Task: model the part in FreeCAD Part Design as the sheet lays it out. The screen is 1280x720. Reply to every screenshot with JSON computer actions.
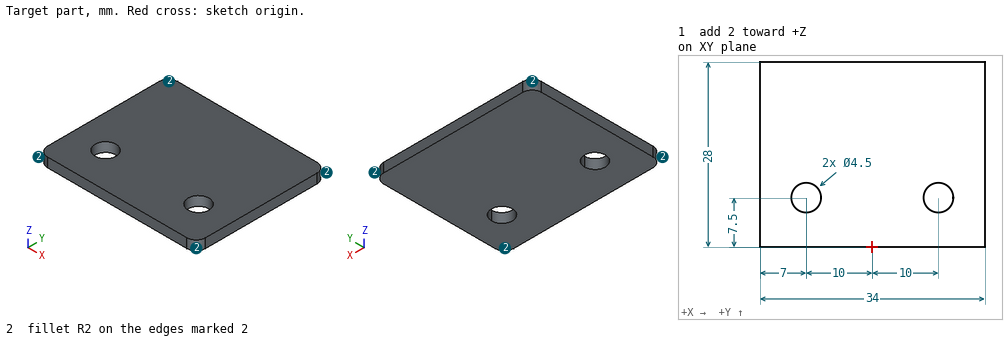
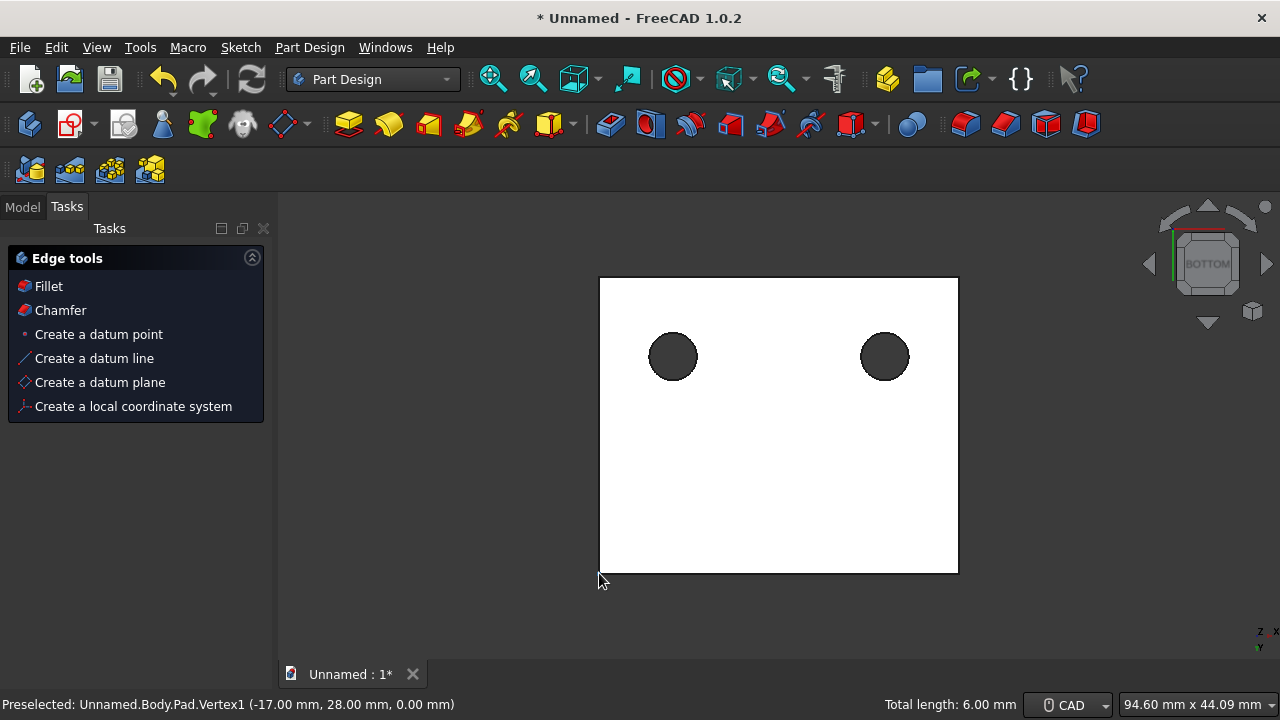
{"action": "key", "text": "4"}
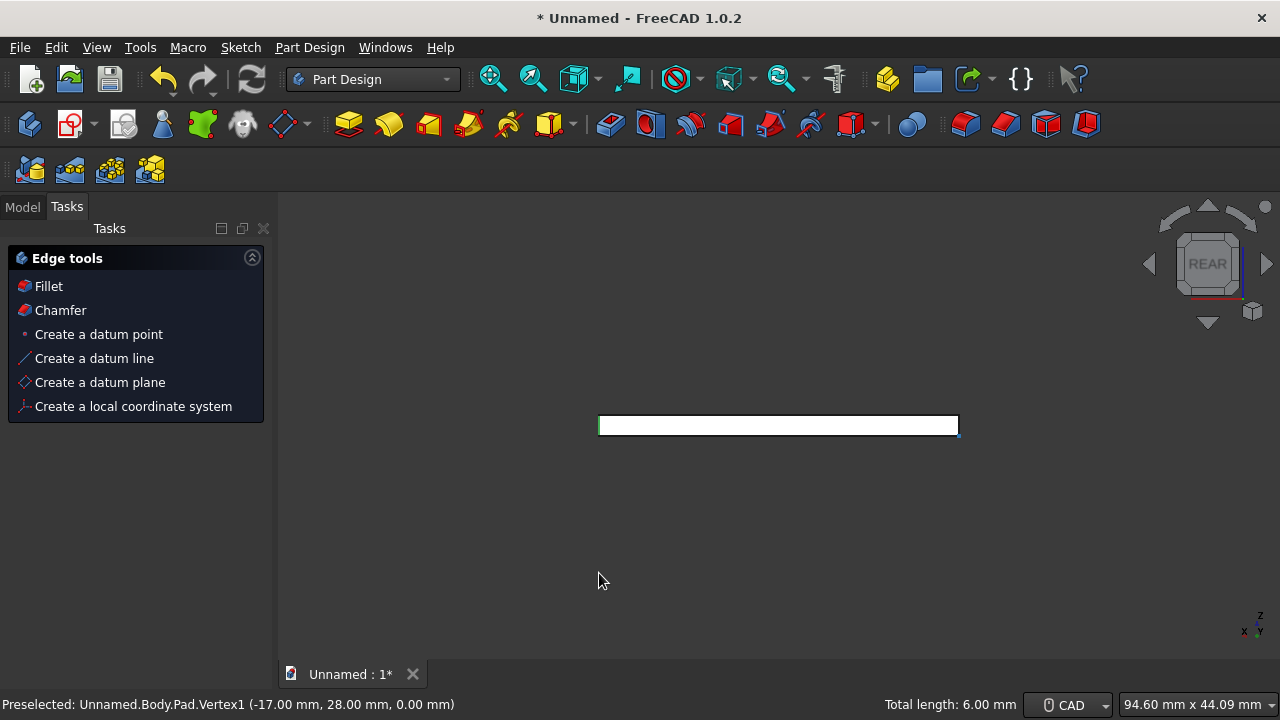
{"action": "key", "text": "v f"}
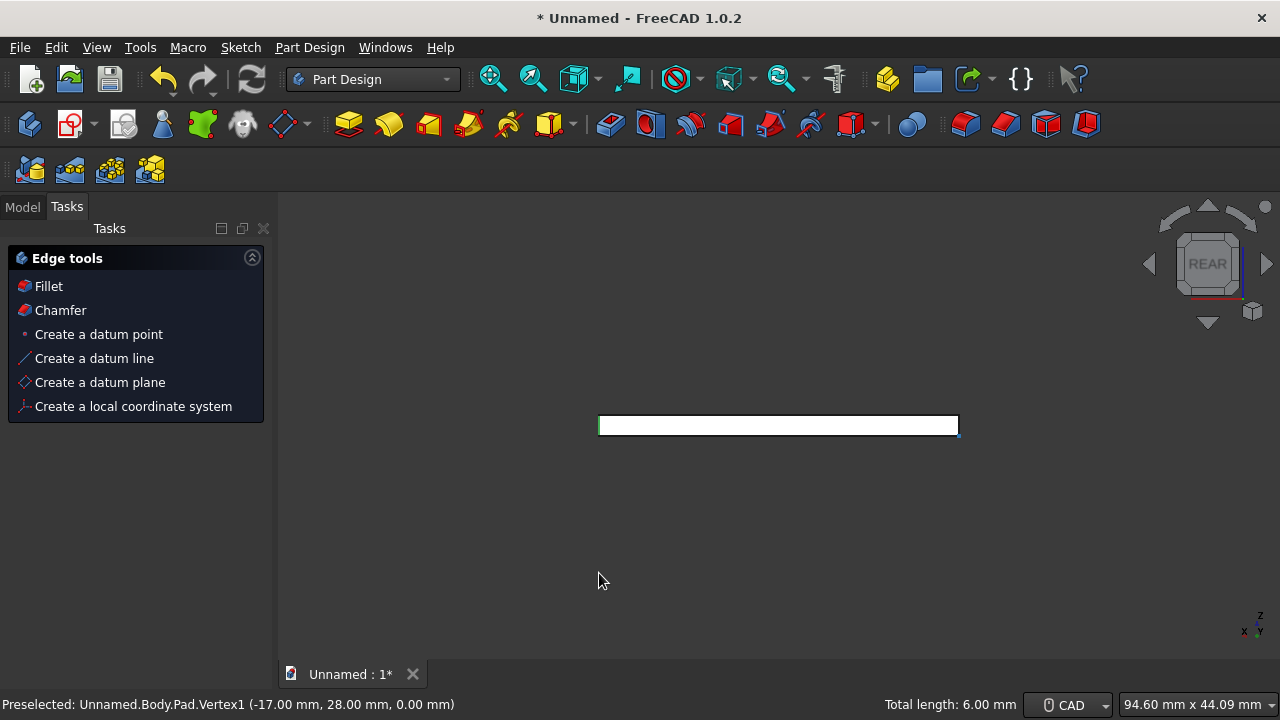
{"action": "left_click", "coordinate": [959, 425], "text": "ctrl"}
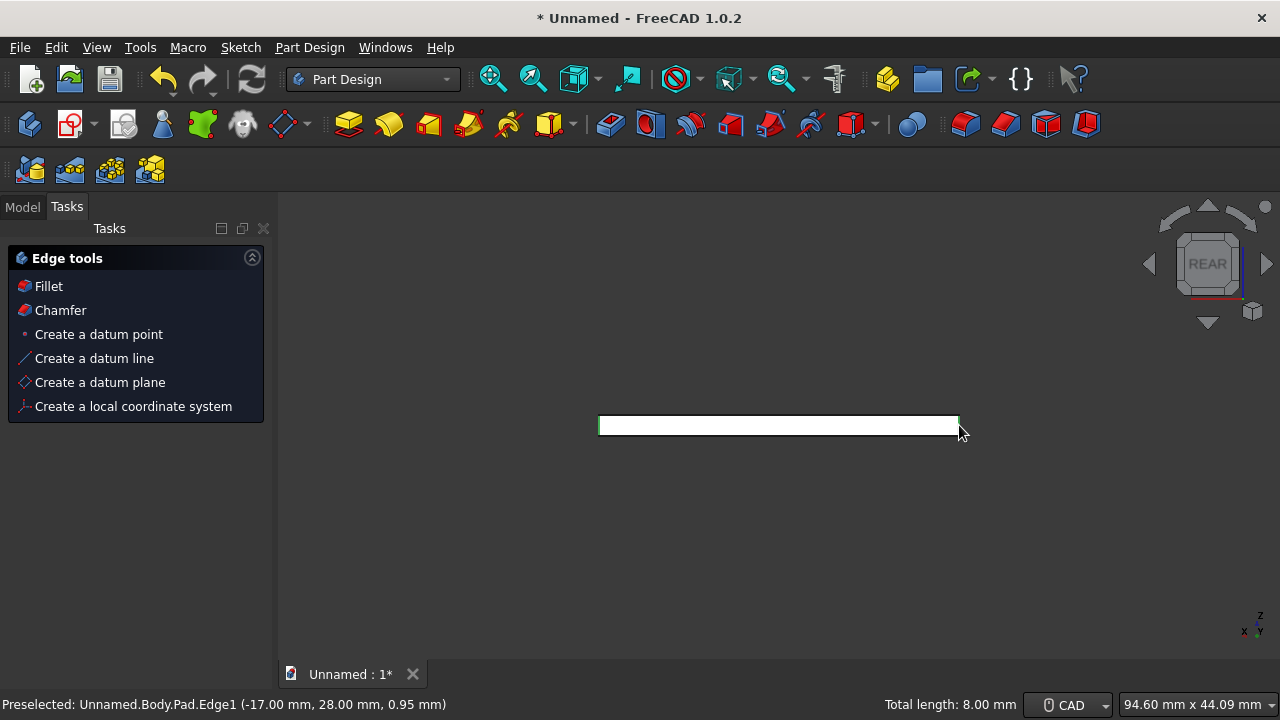
{"action": "left_click", "coordinate": [966, 124]}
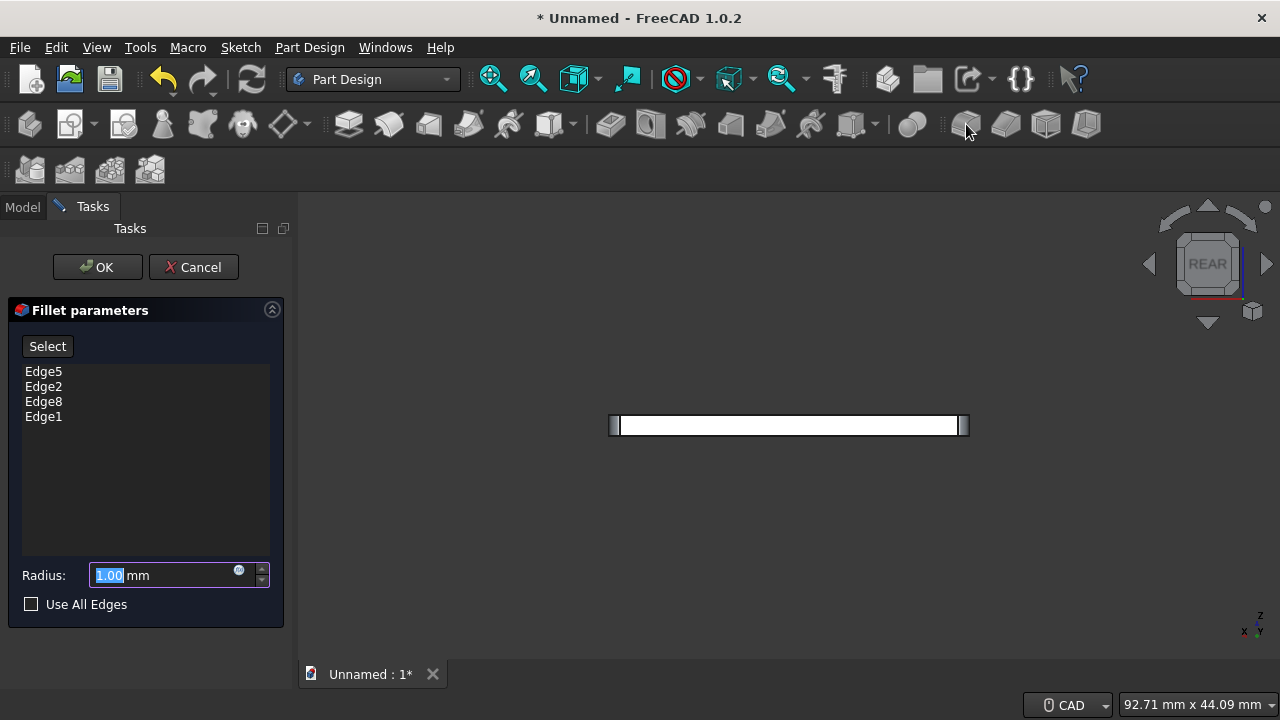
{"action": "type", "text": "2"}
{"action": "key", "text": "Tab"}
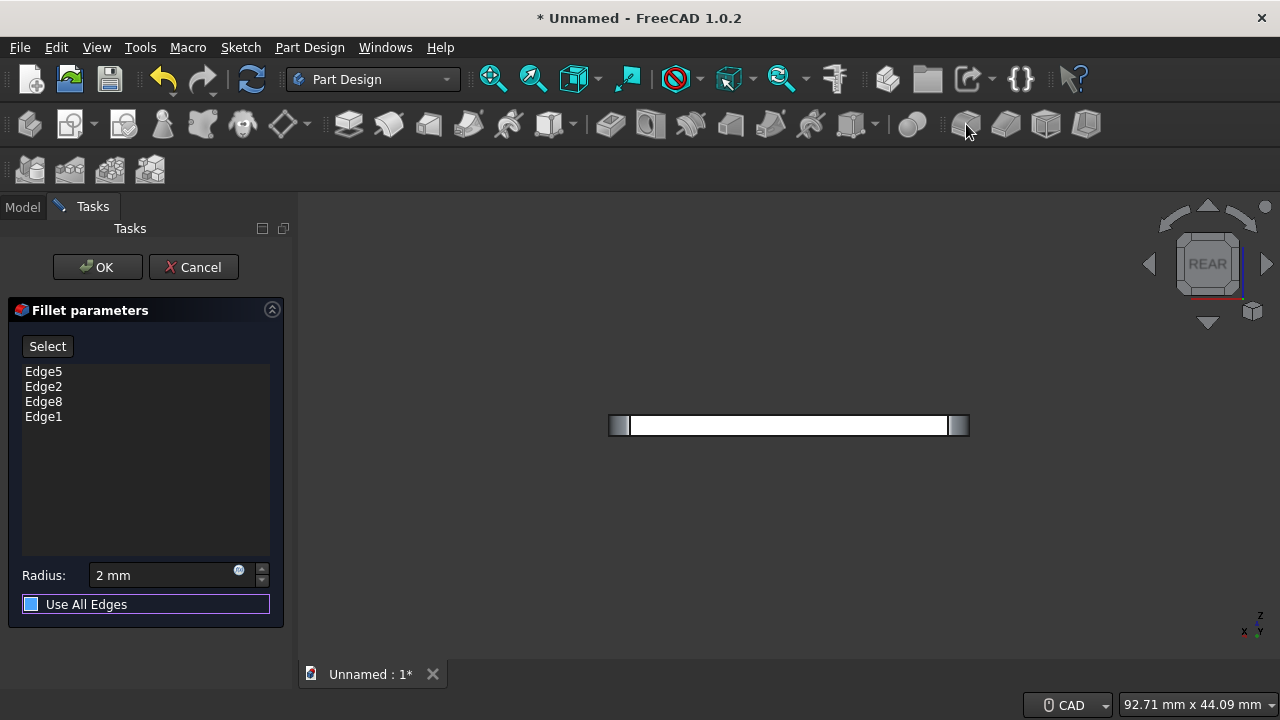
{"action": "left_click", "coordinate": [98, 267]}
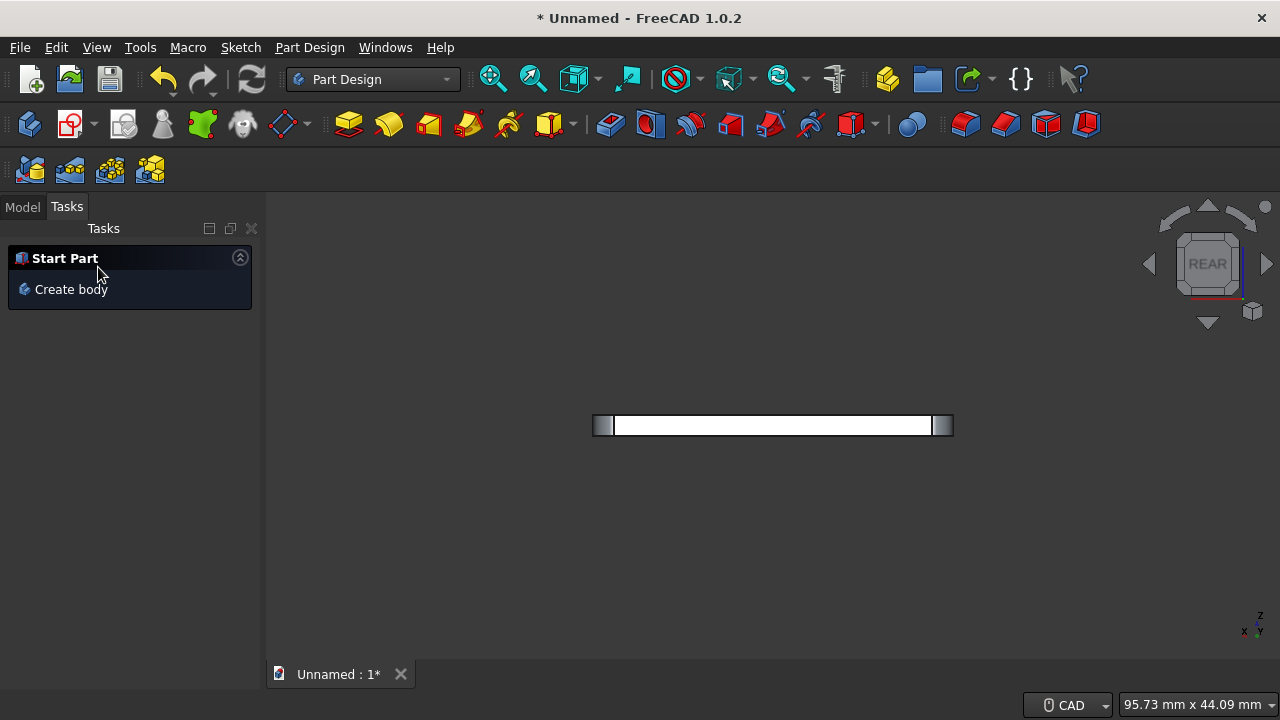
{"action": "key", "text": "0"}